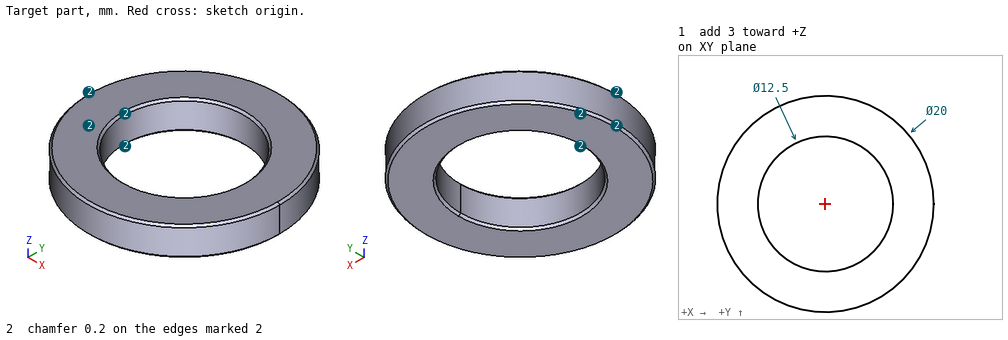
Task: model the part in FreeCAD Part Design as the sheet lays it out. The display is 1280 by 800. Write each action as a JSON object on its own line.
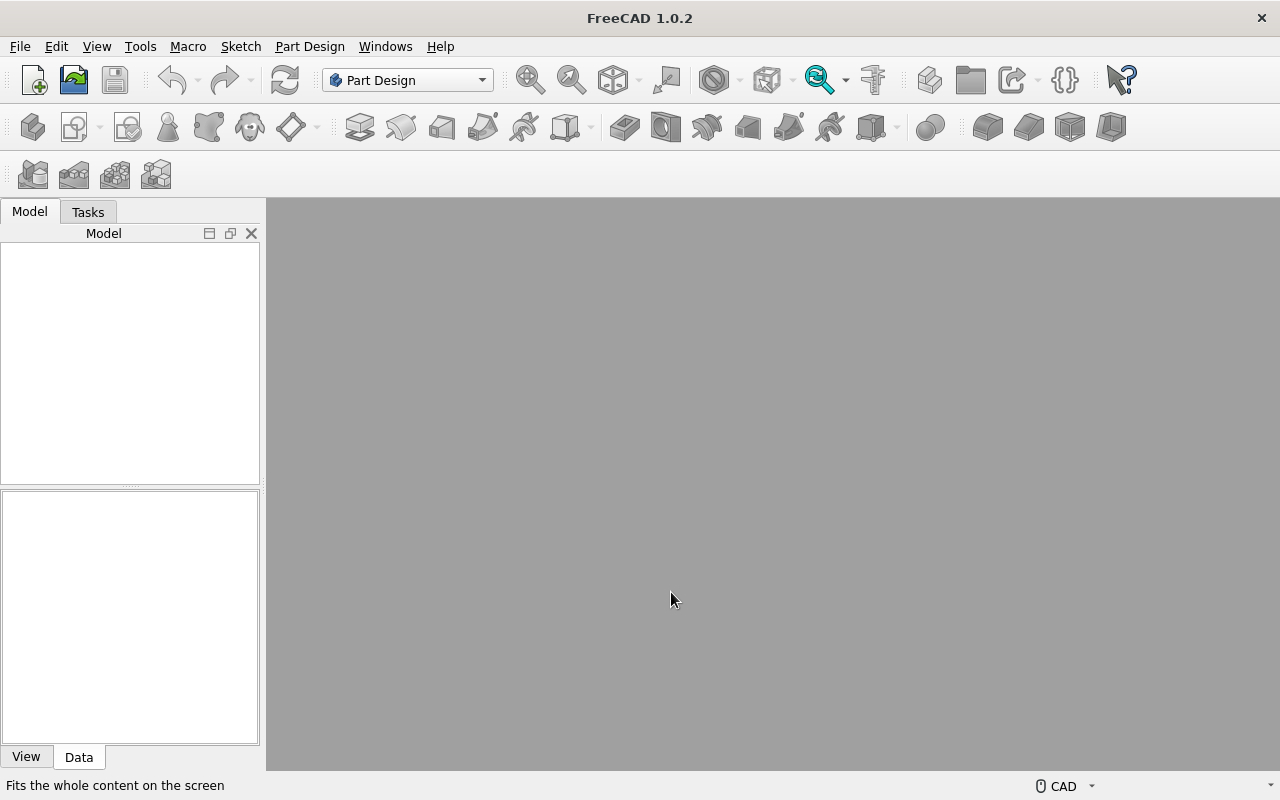
{"action": "left_click", "coordinate": [33, 80]}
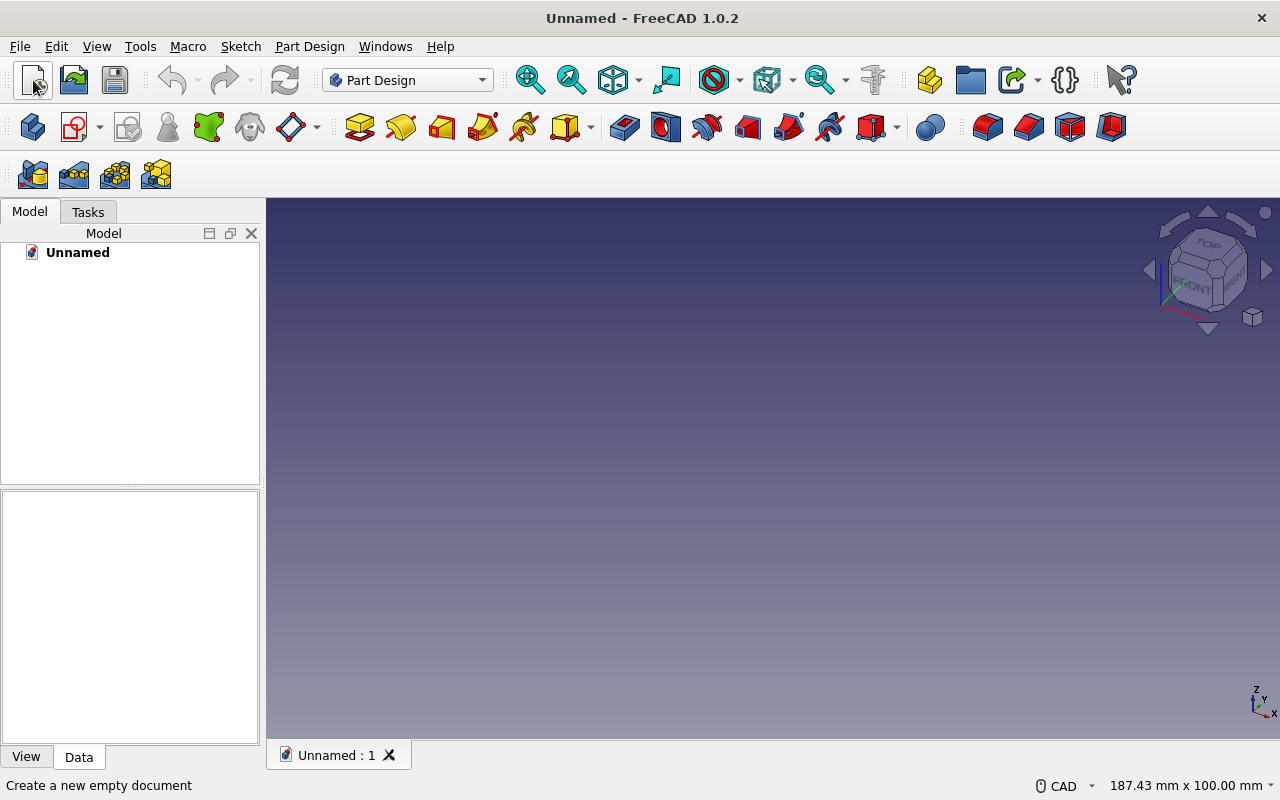
{"action": "left_click", "coordinate": [74, 128]}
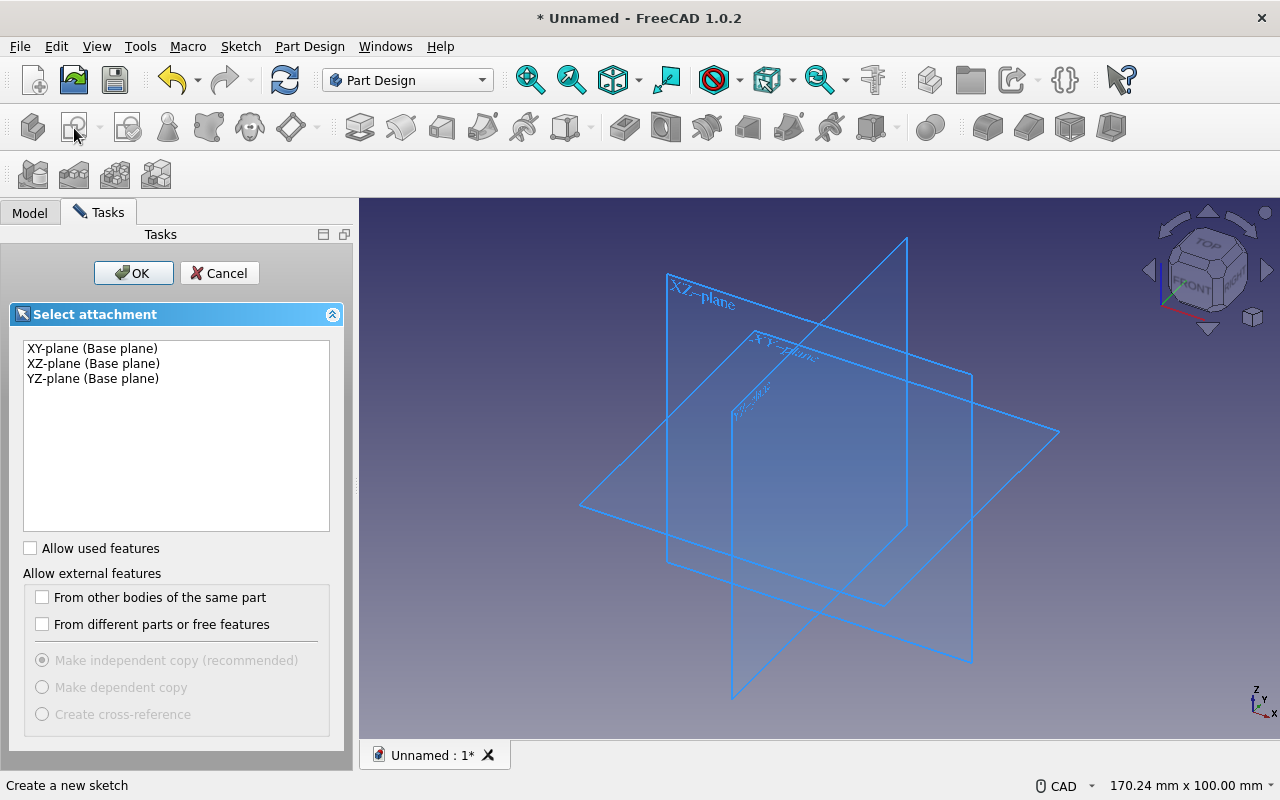
{"action": "left_click", "coordinate": [84, 348]}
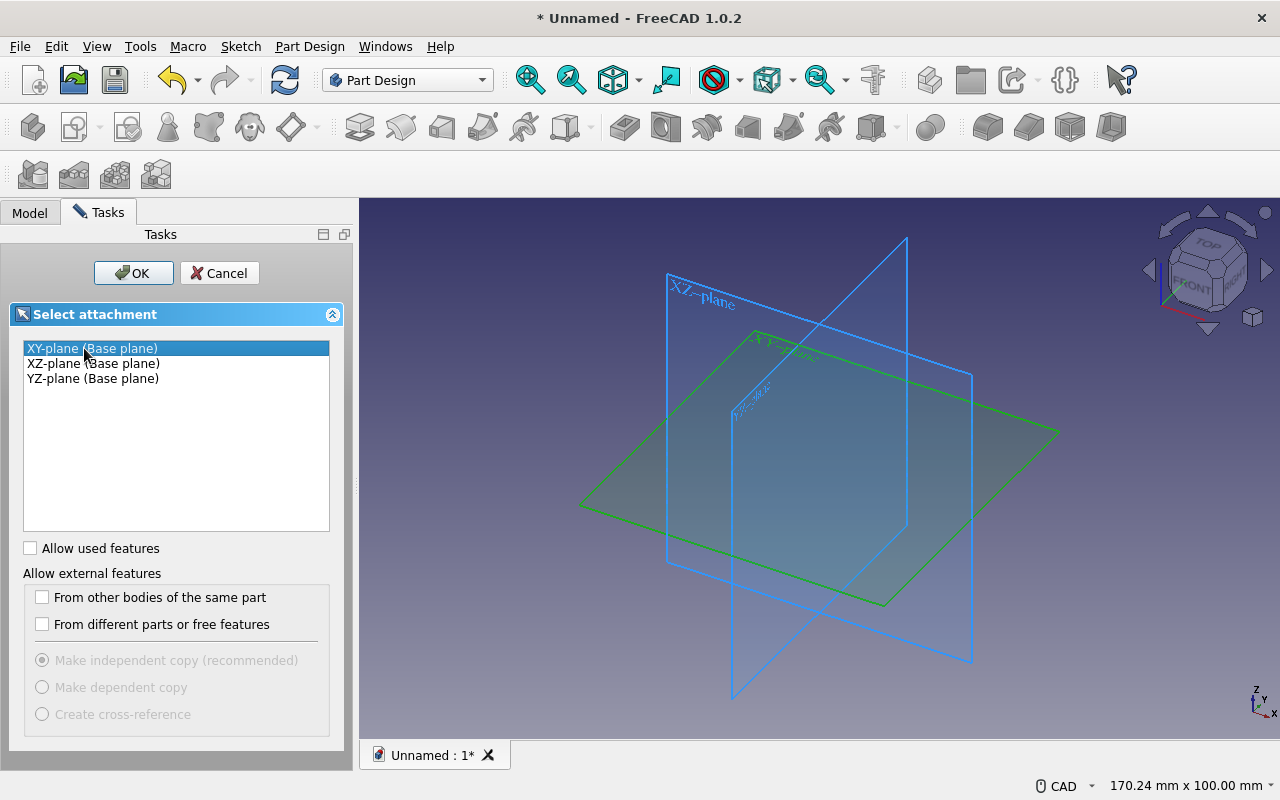
{"action": "left_click", "coordinate": [134, 273]}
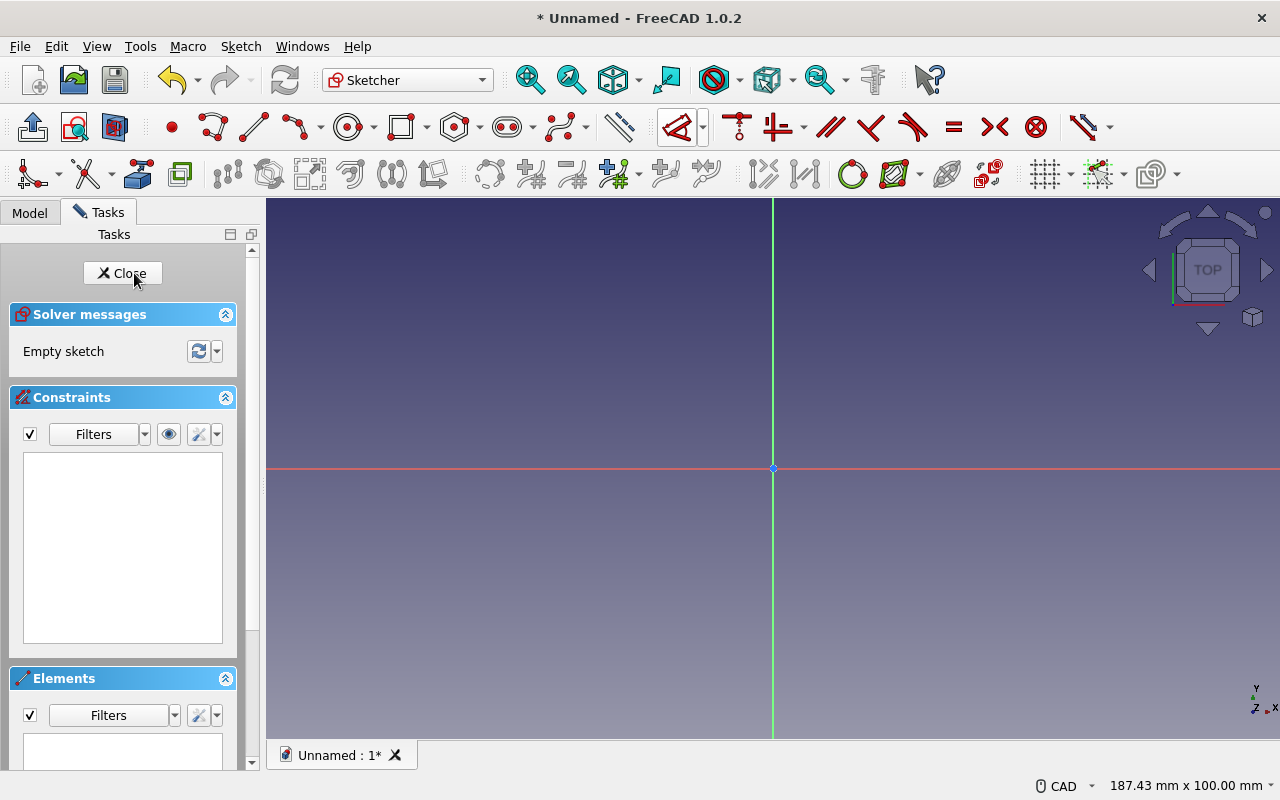
{"action": "scroll", "coordinate": [803, 468], "scroll_direction": "up", "scroll_amount": 6}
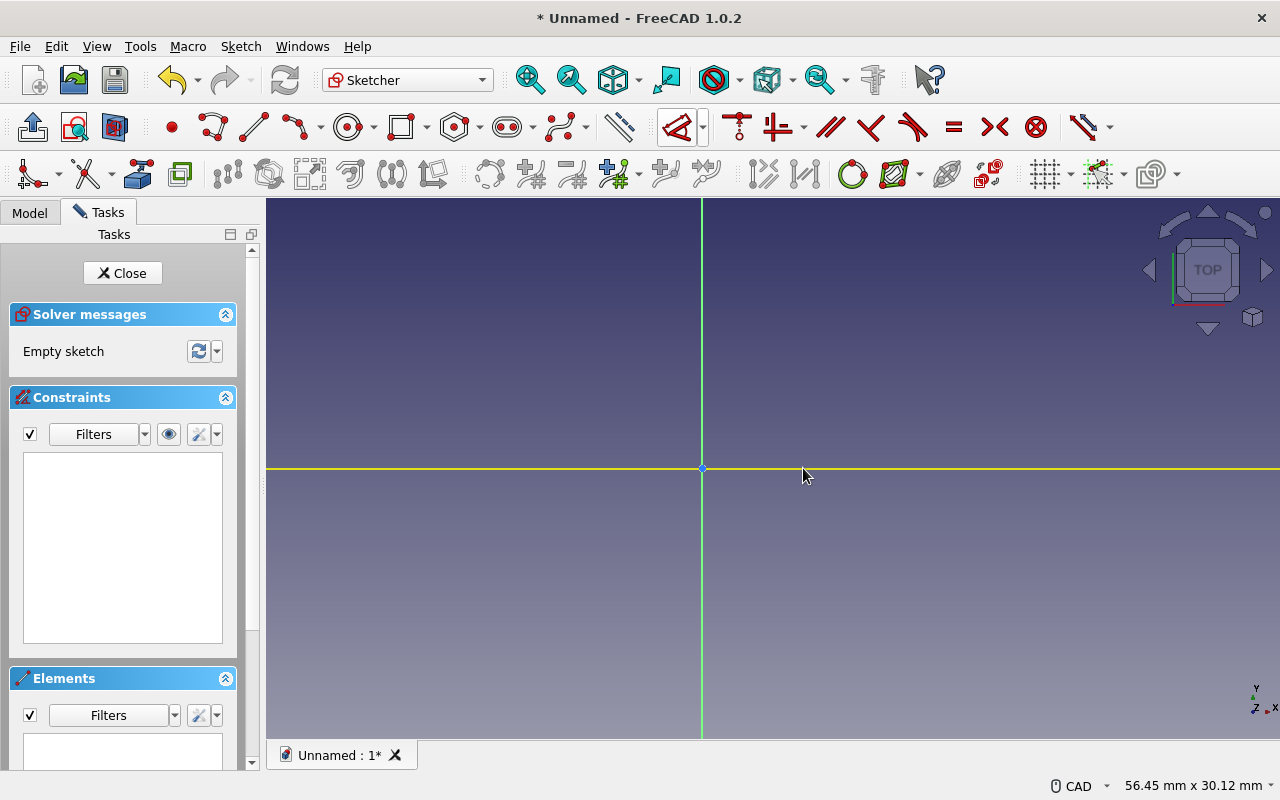
{"action": "left_click", "coordinate": [348, 128]}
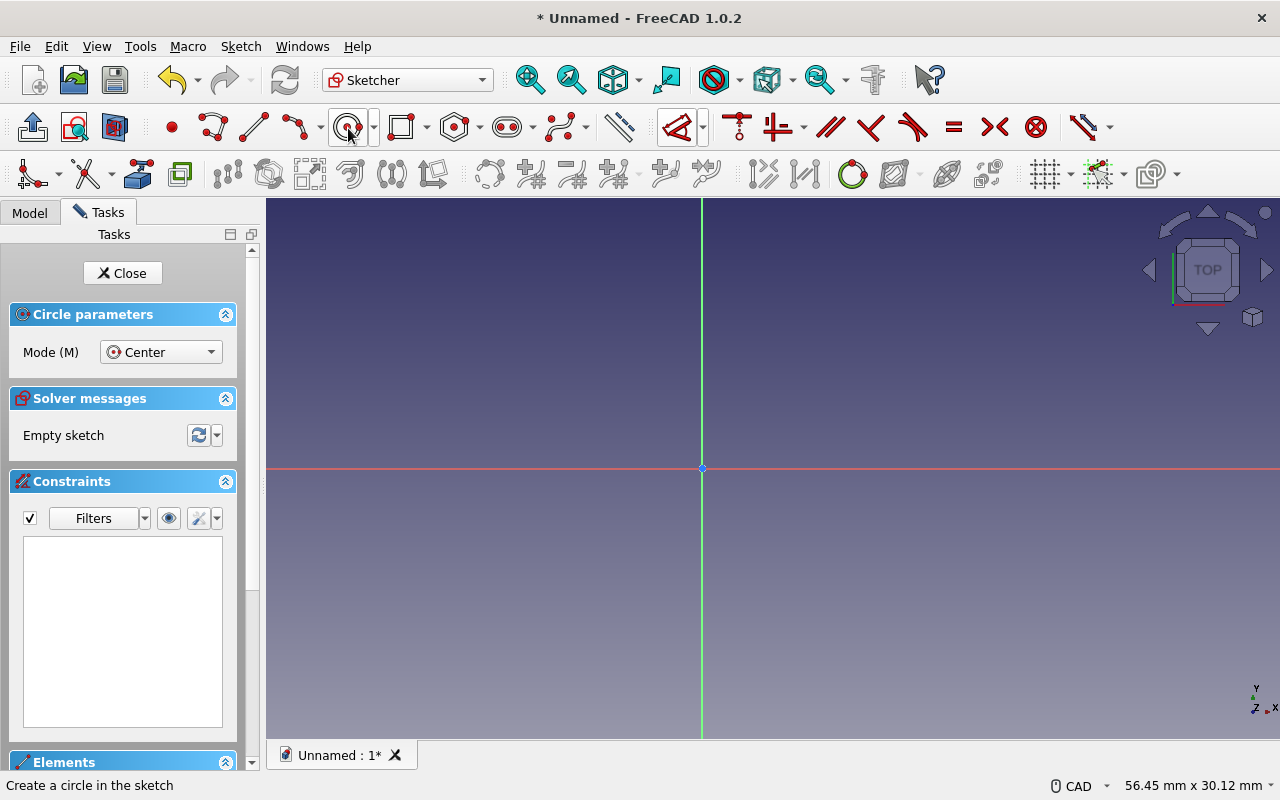
{"action": "left_click", "coordinate": [702, 468]}
{"action": "left_click", "coordinate": [829, 341]}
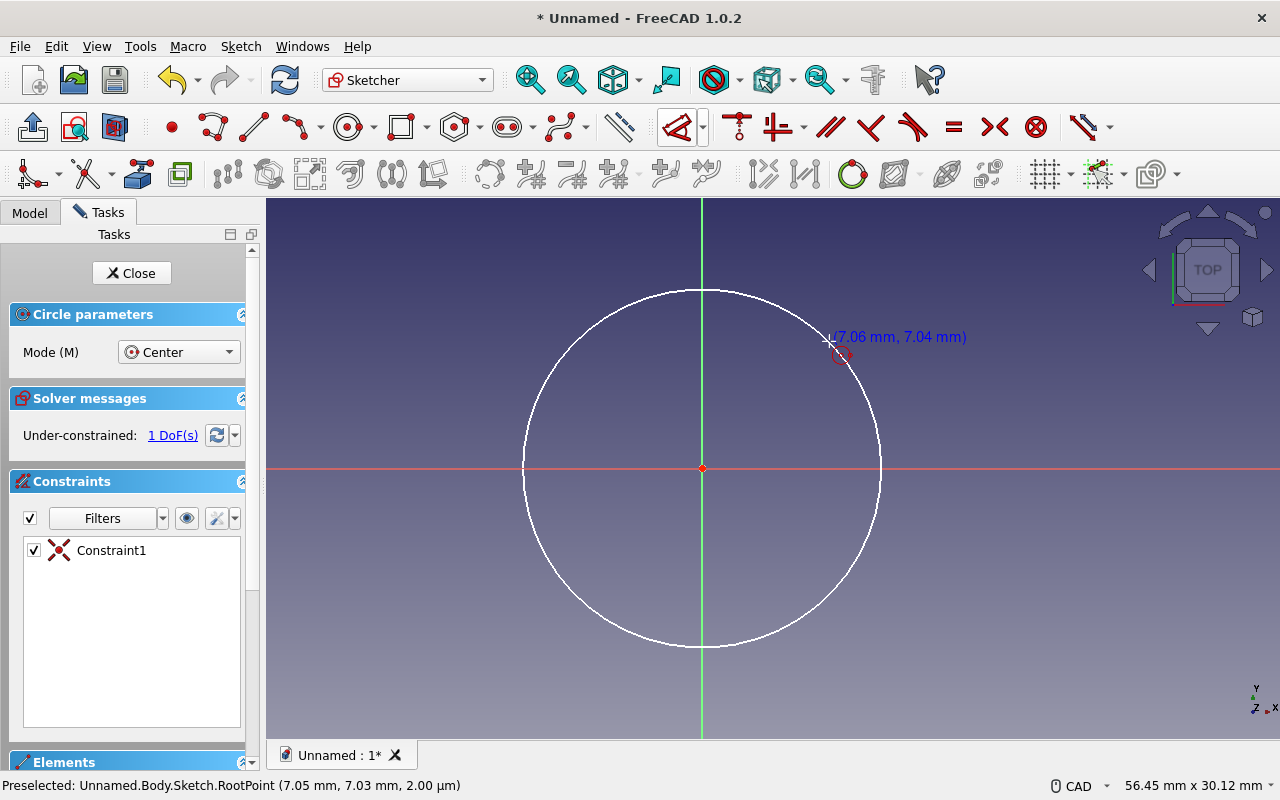
{"action": "left_click", "coordinate": [702, 468]}
{"action": "left_click", "coordinate": [782, 389]}
{"action": "key", "text": "Escape"}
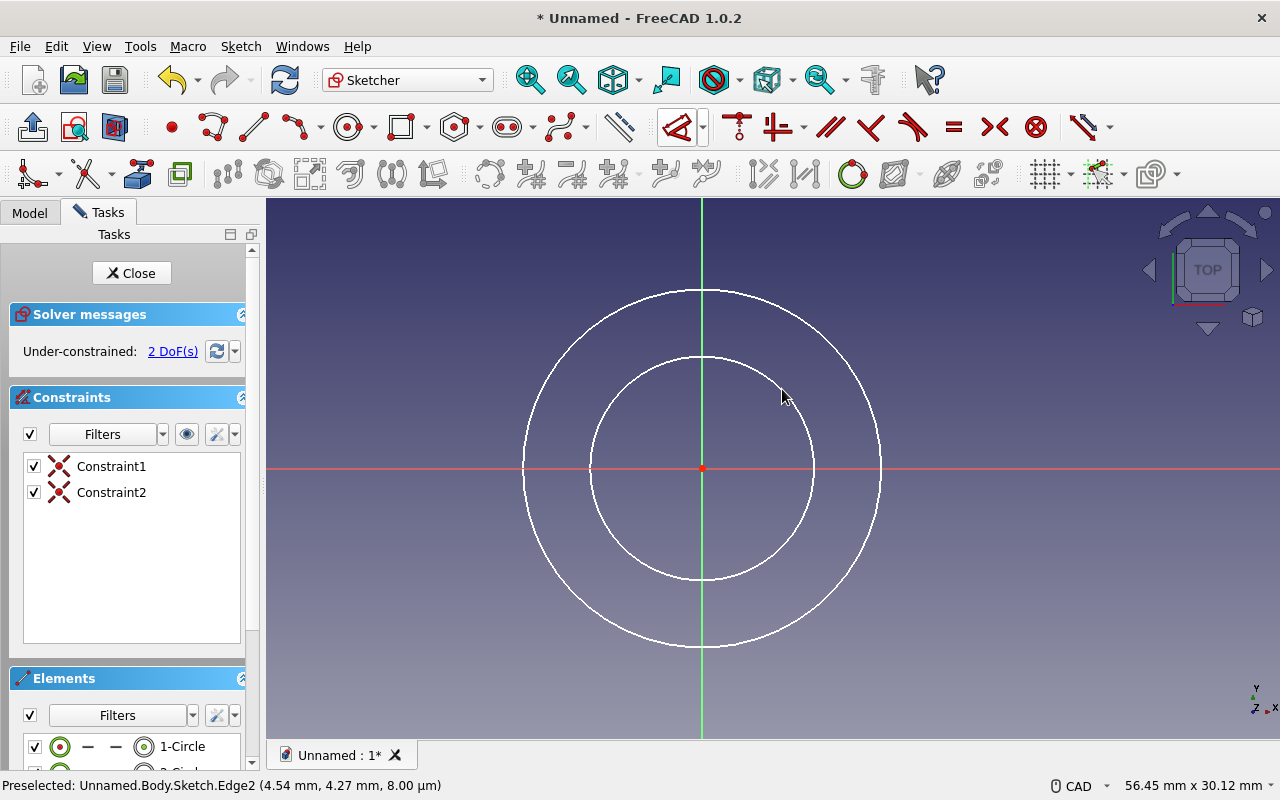
{"action": "left_click", "coordinate": [676, 128]}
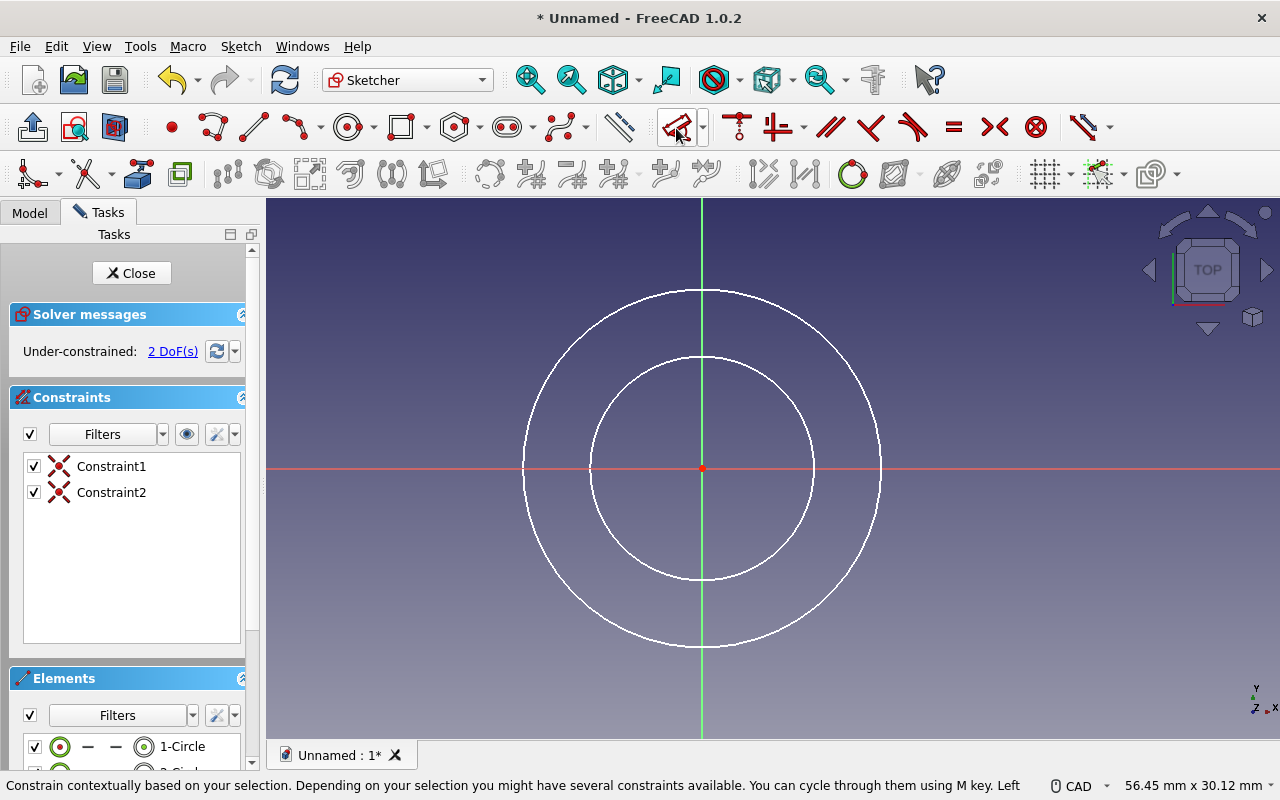
{"action": "left_click", "coordinate": [828, 341]}
{"action": "left_click", "coordinate": [850, 318]}